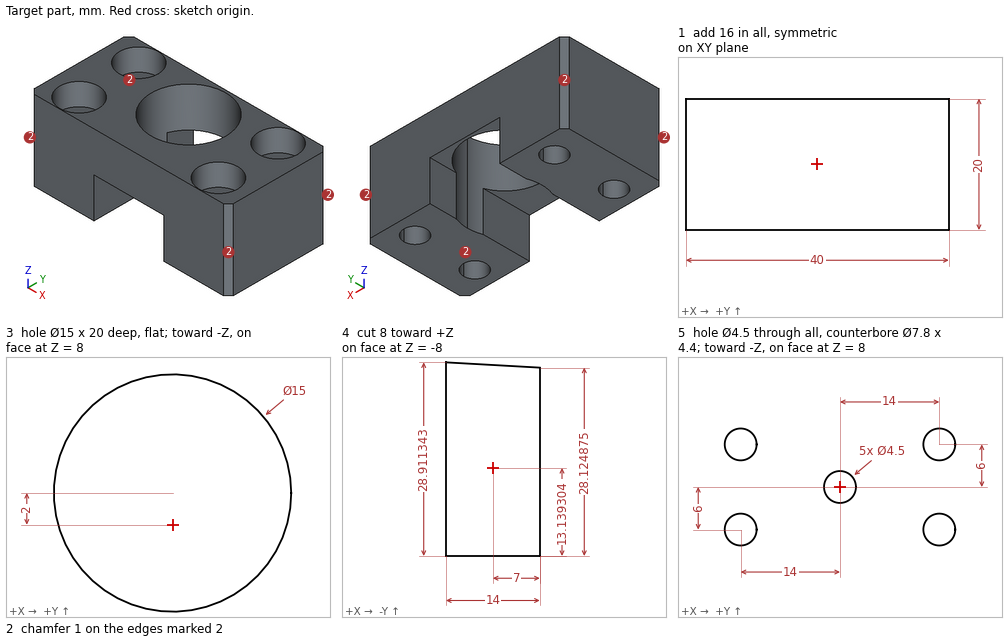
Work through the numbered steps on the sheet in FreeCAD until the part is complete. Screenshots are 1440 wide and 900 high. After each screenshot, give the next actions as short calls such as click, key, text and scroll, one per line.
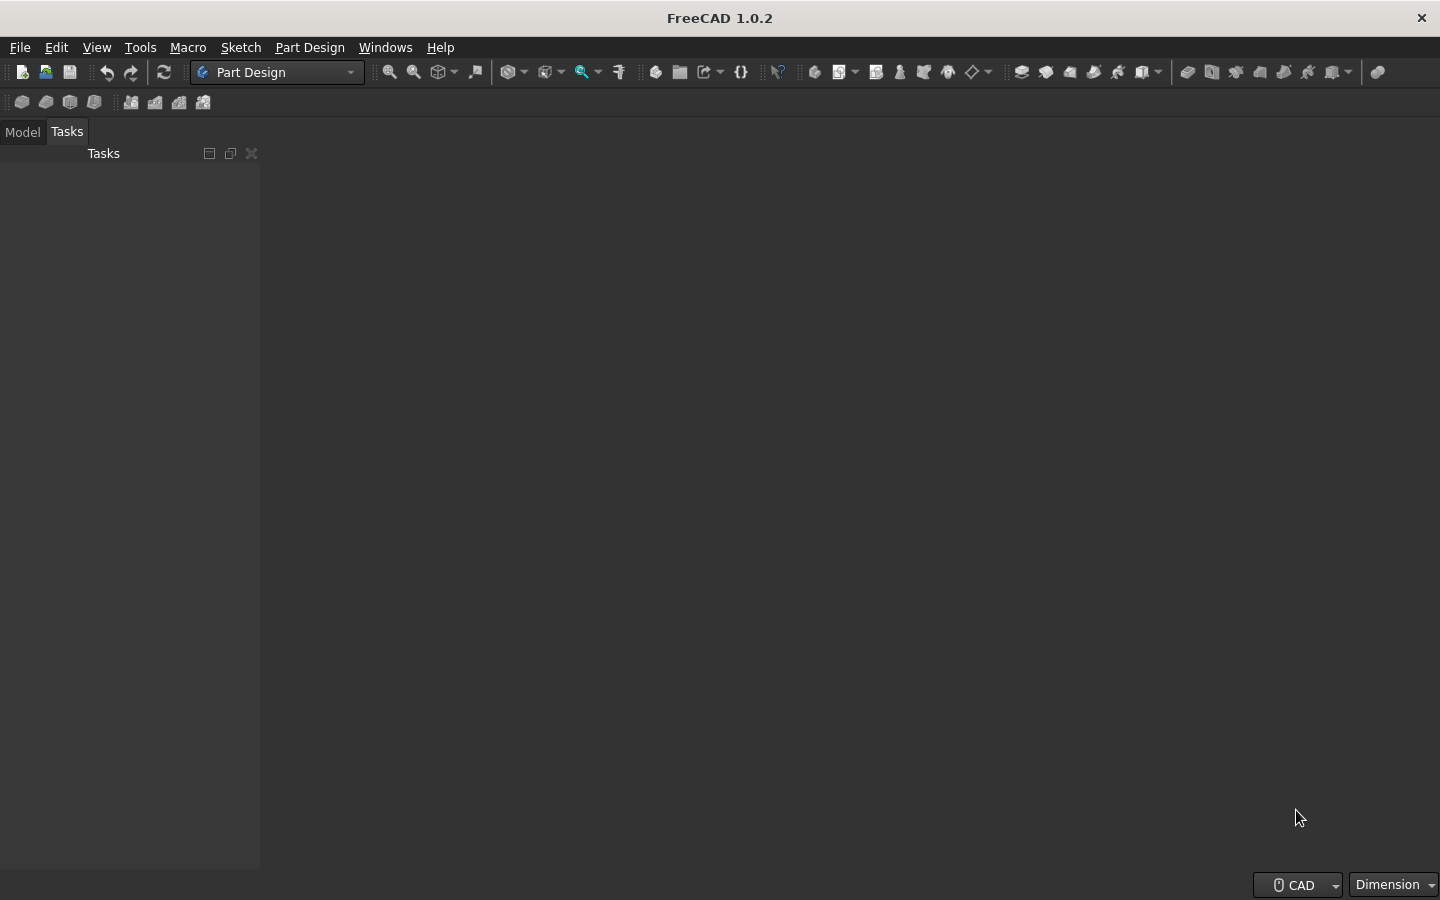
key(ctrl+n)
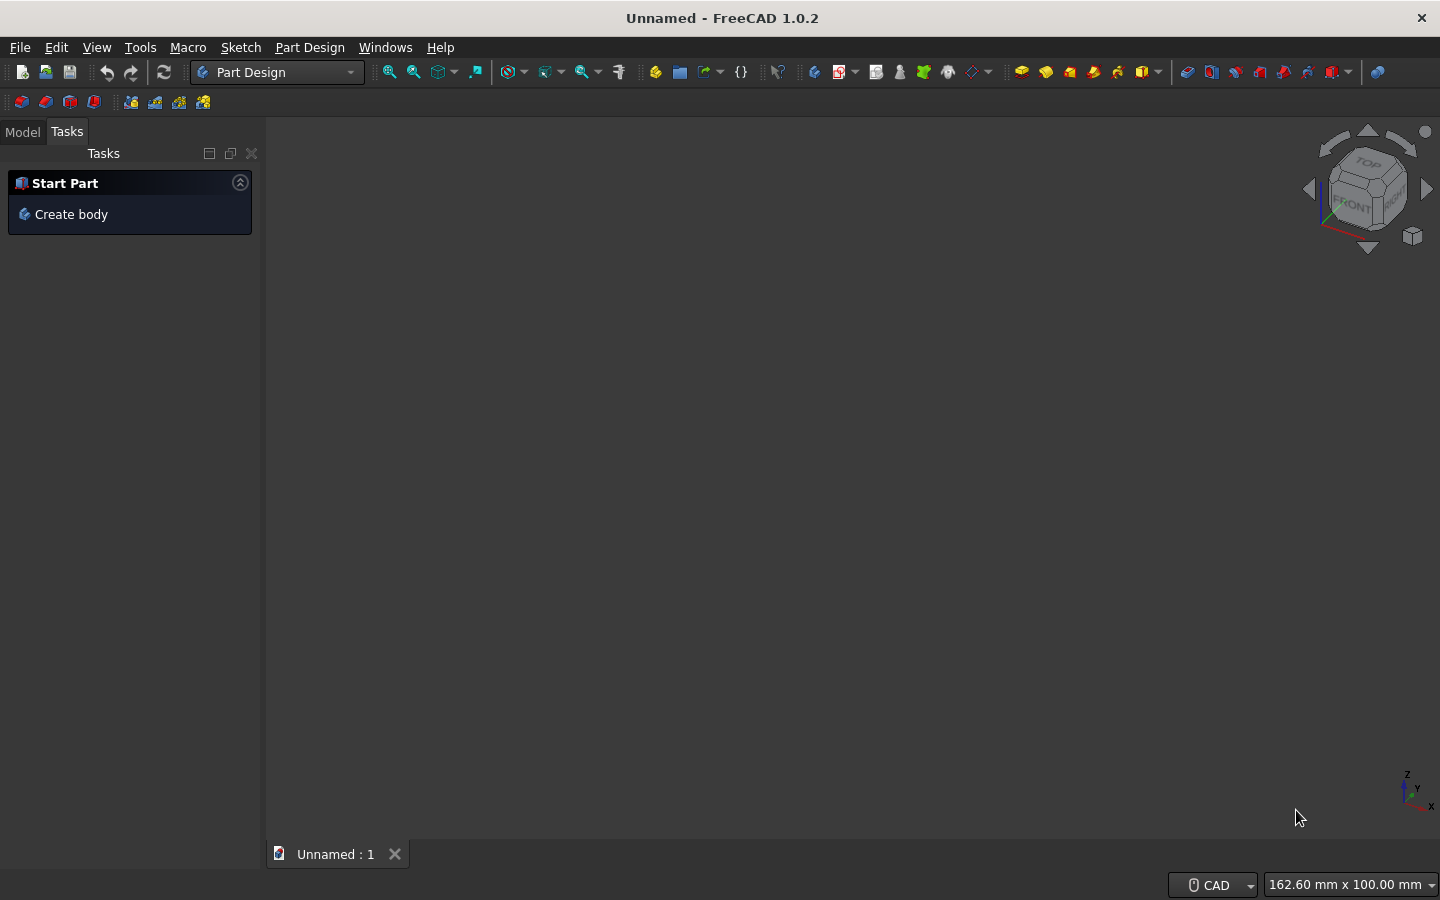
click(840, 72)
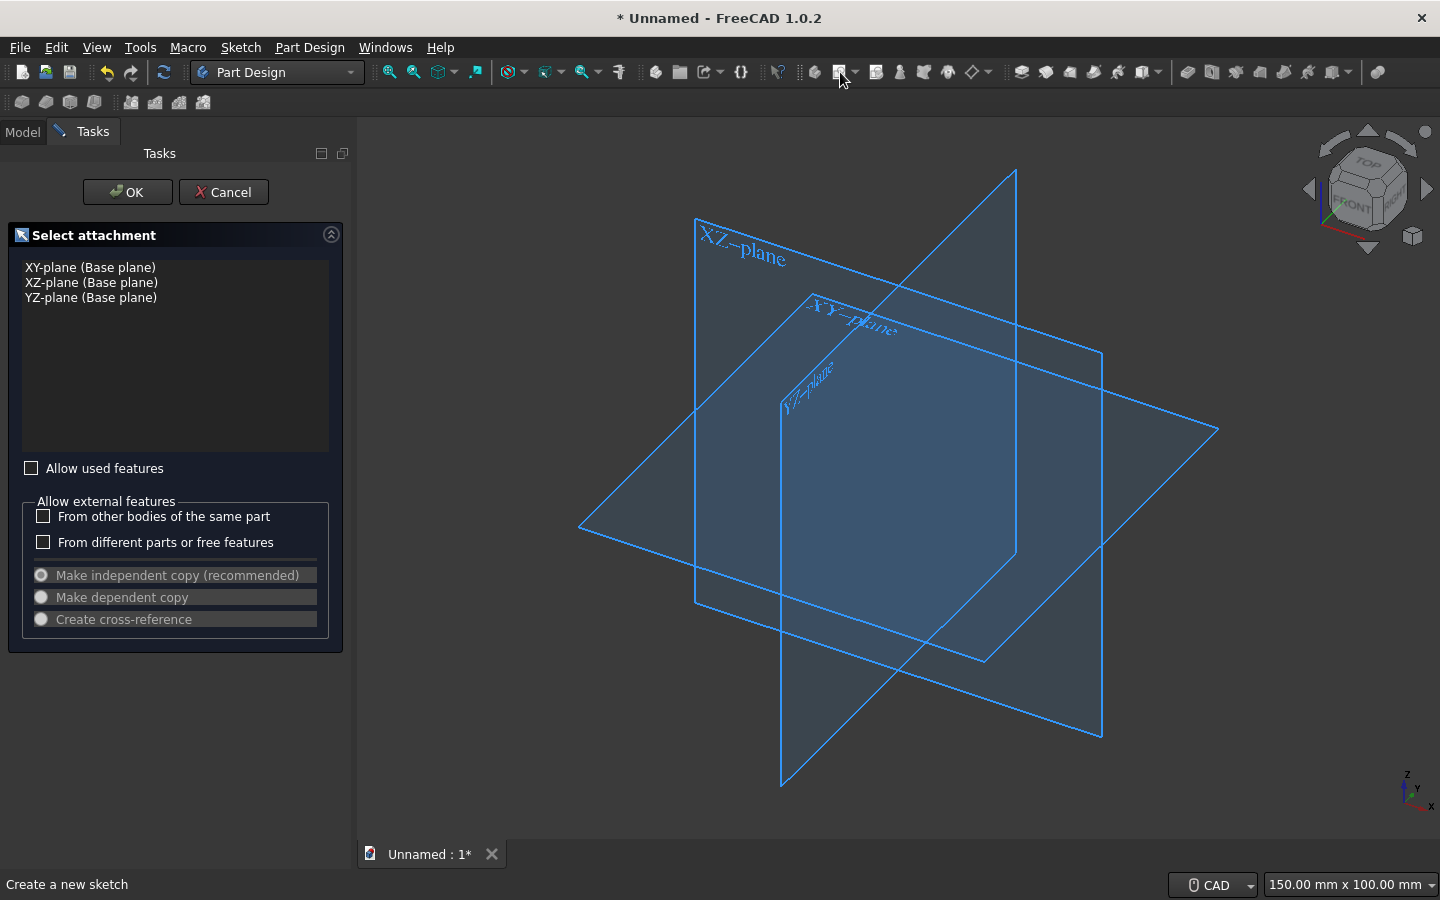
click(82, 268)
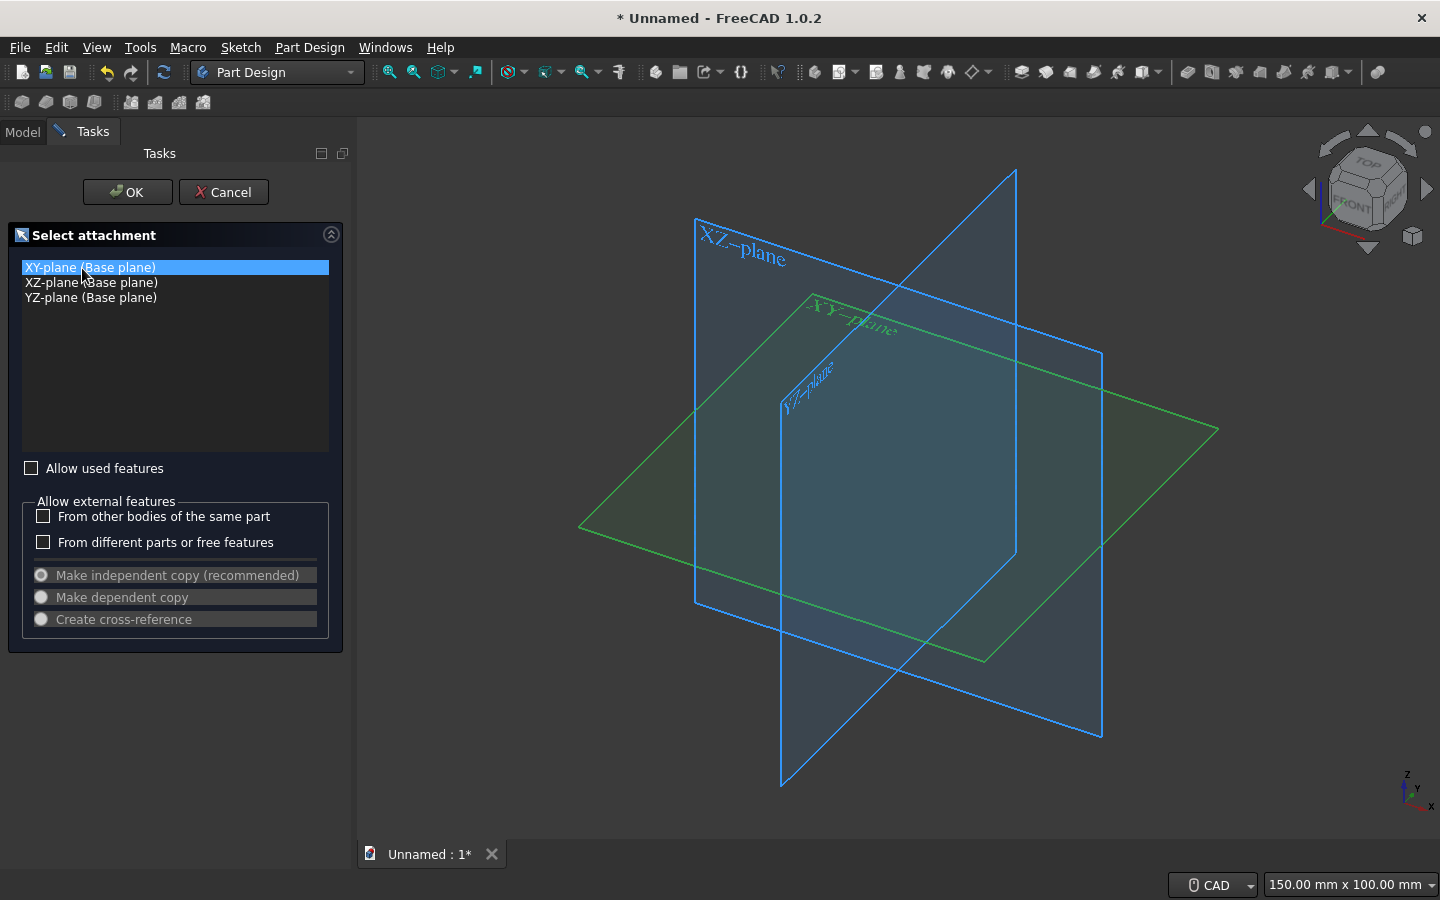
click(128, 192)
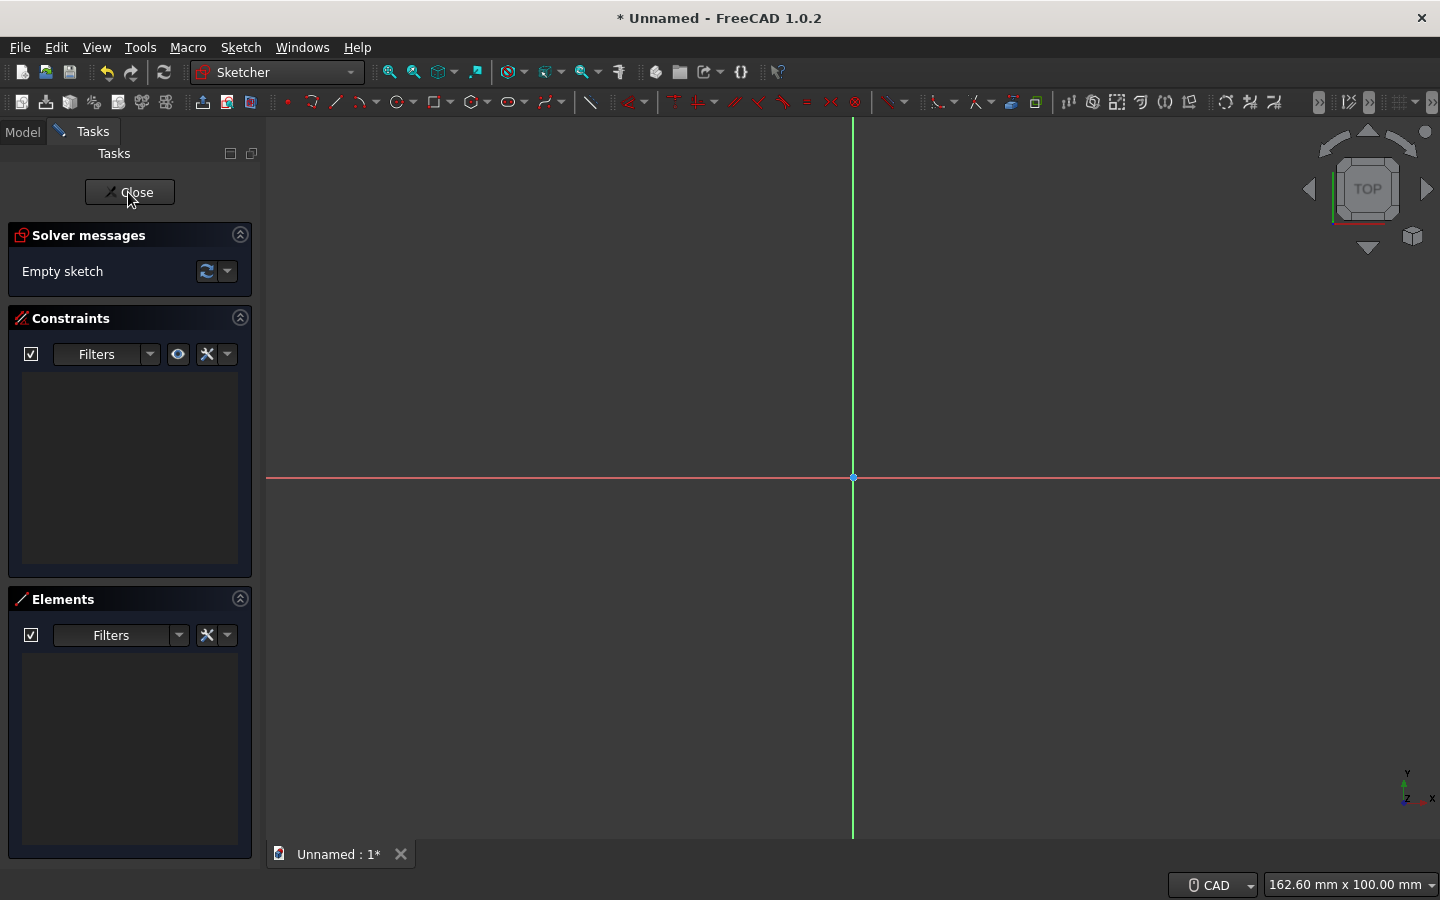
scroll(909, 478, up, 4)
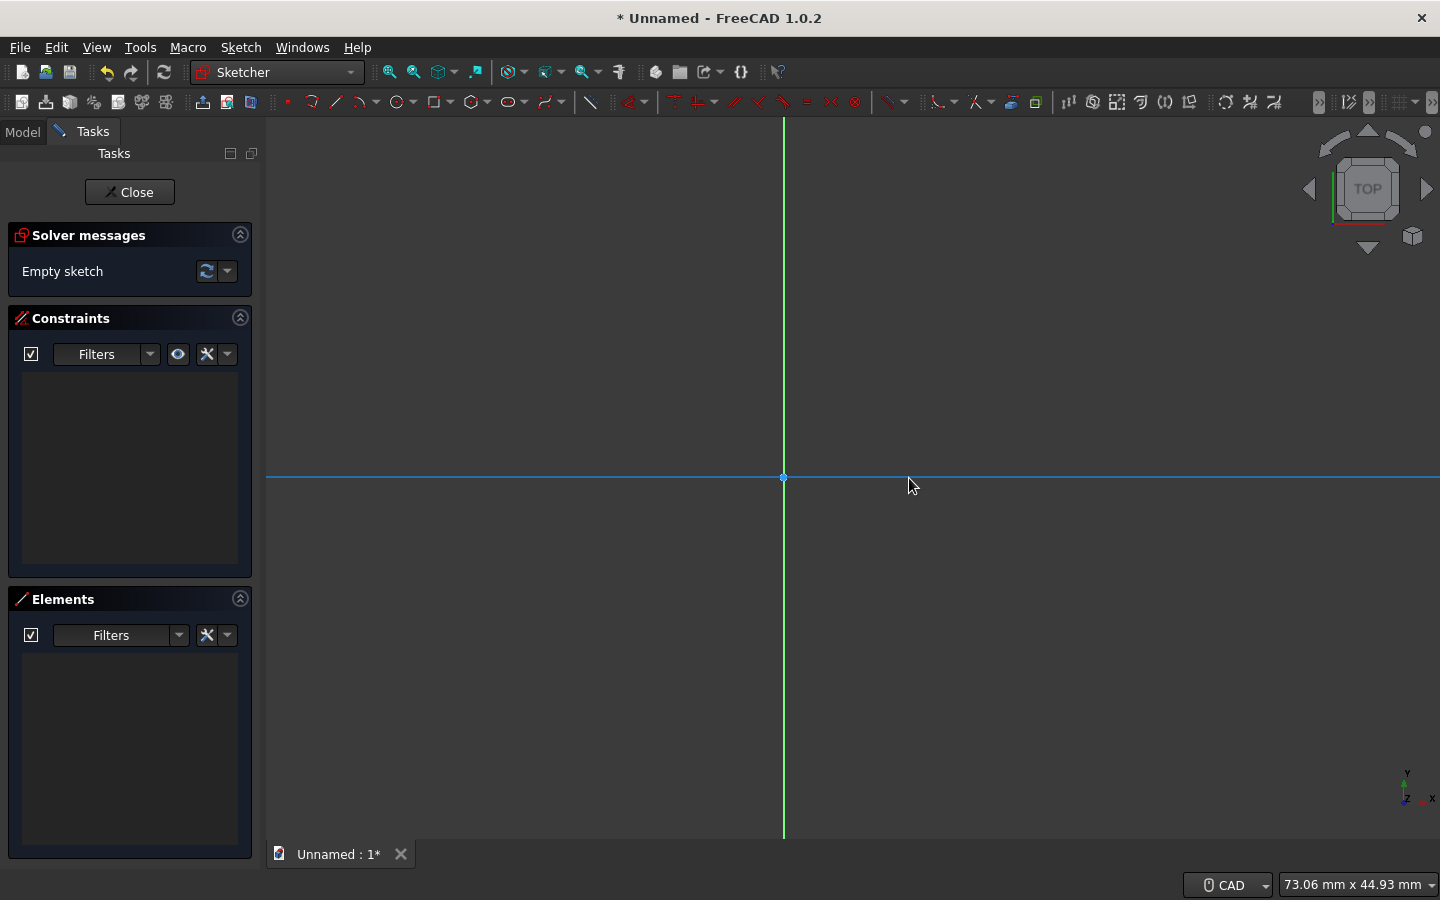
key(g)
key(v)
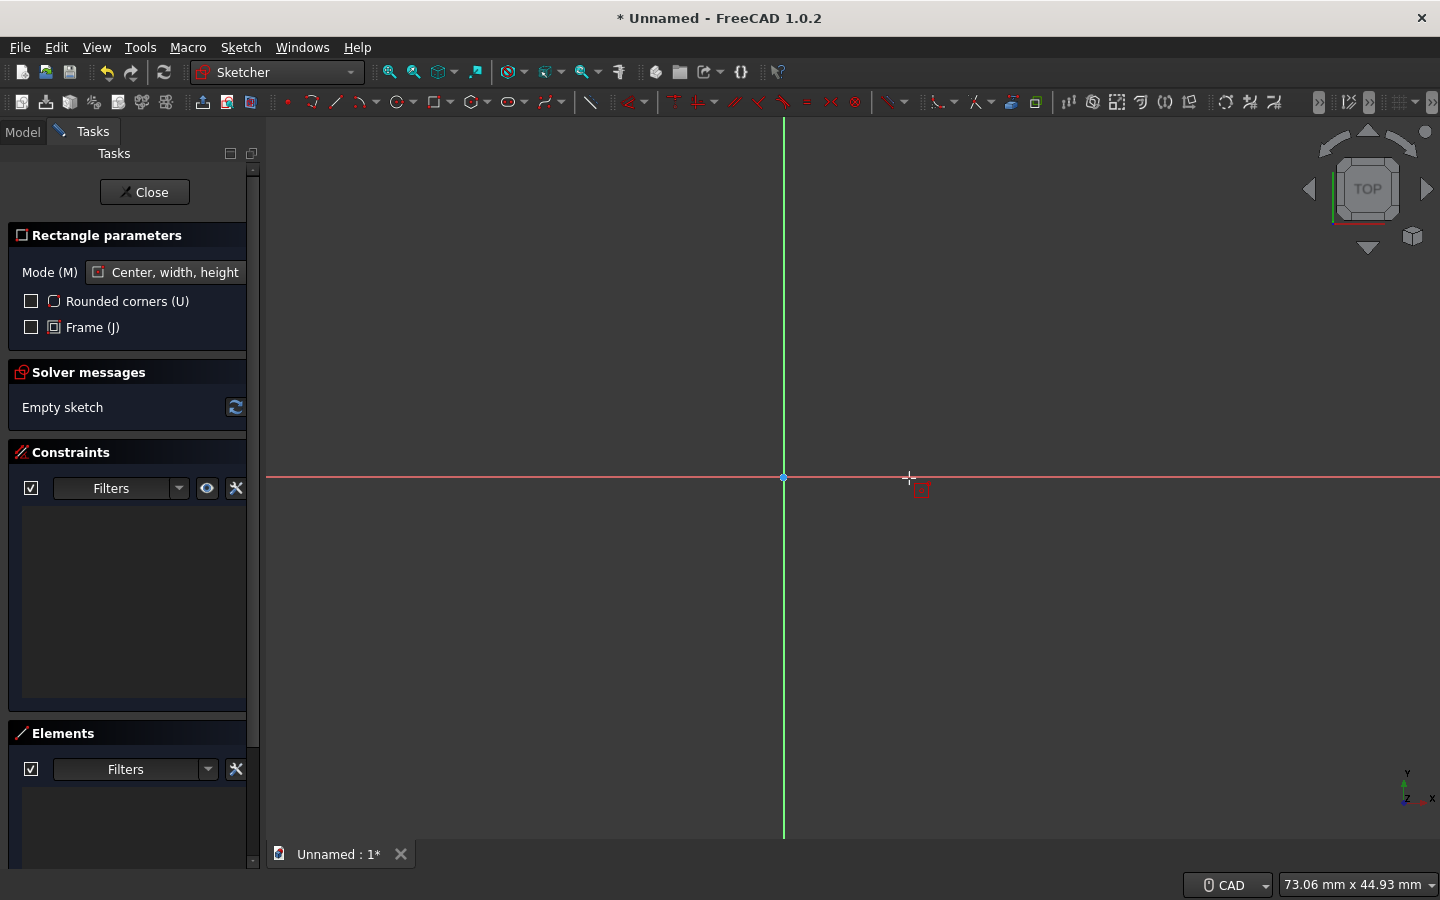
click(784, 477)
click(1105, 317)
key(Escape)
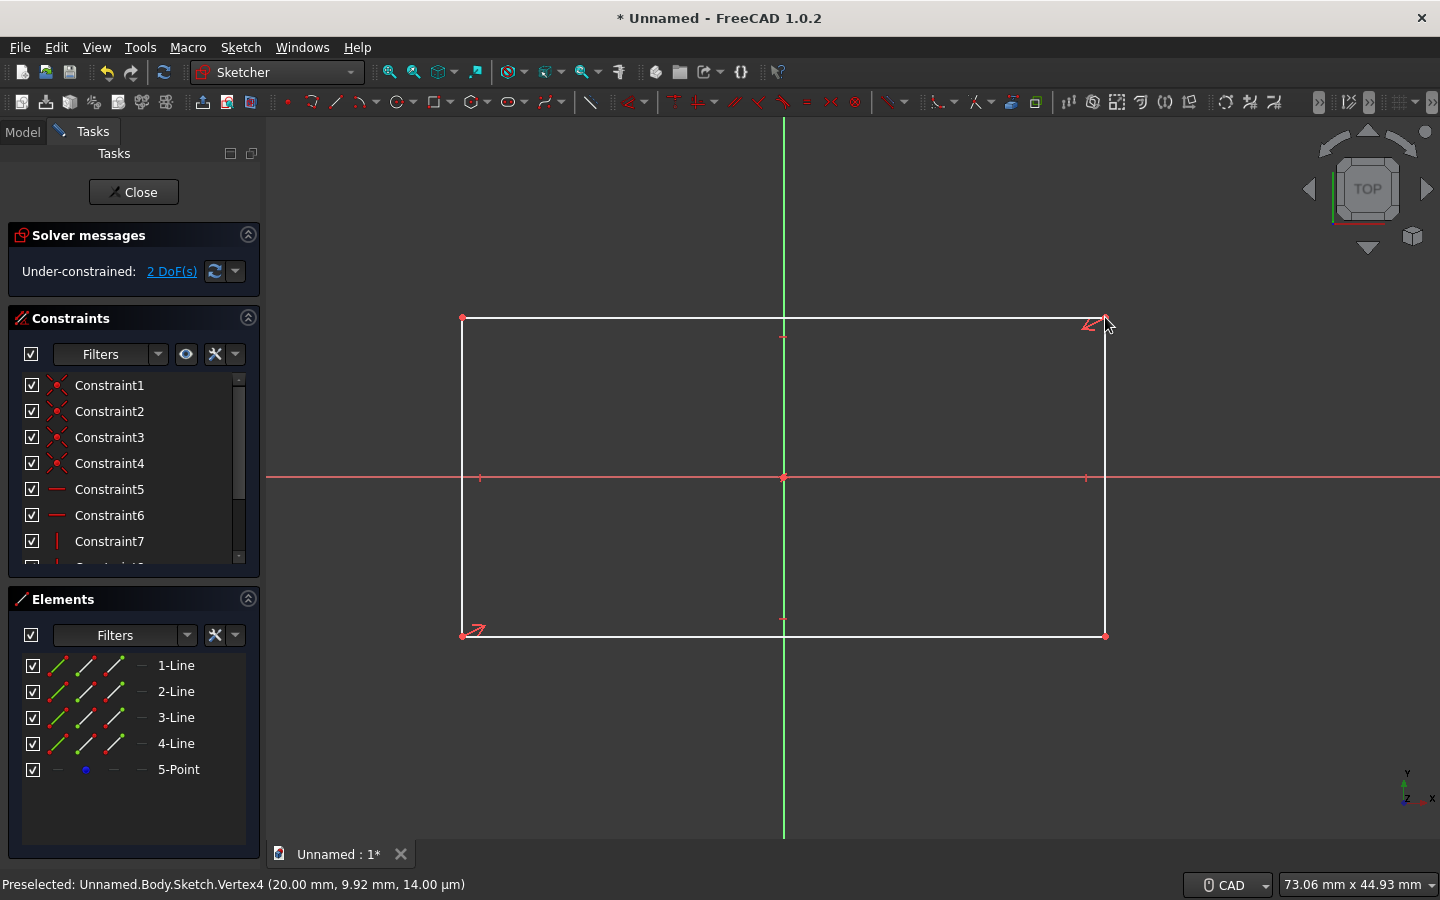
key(d)